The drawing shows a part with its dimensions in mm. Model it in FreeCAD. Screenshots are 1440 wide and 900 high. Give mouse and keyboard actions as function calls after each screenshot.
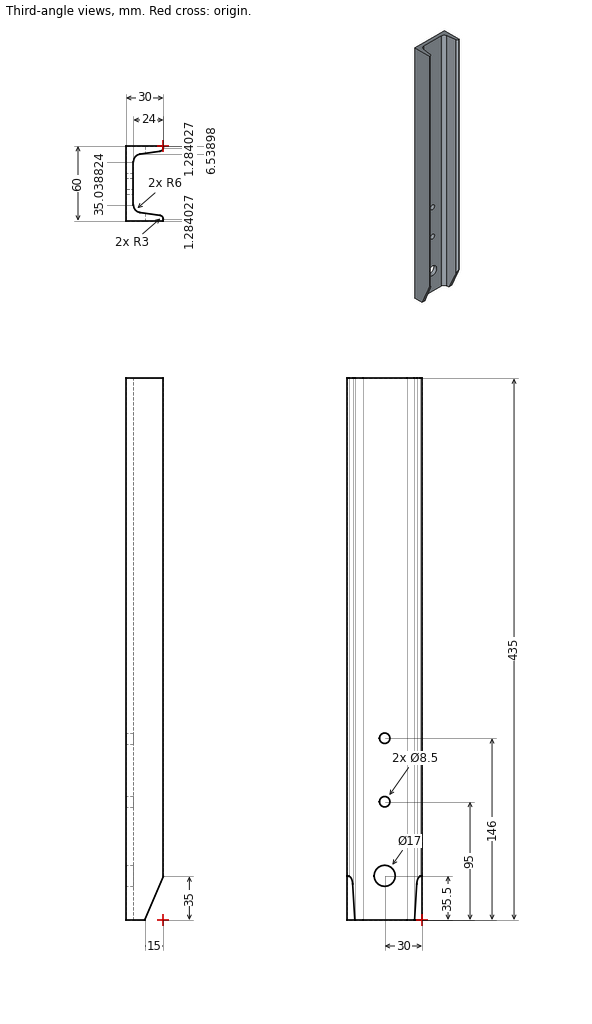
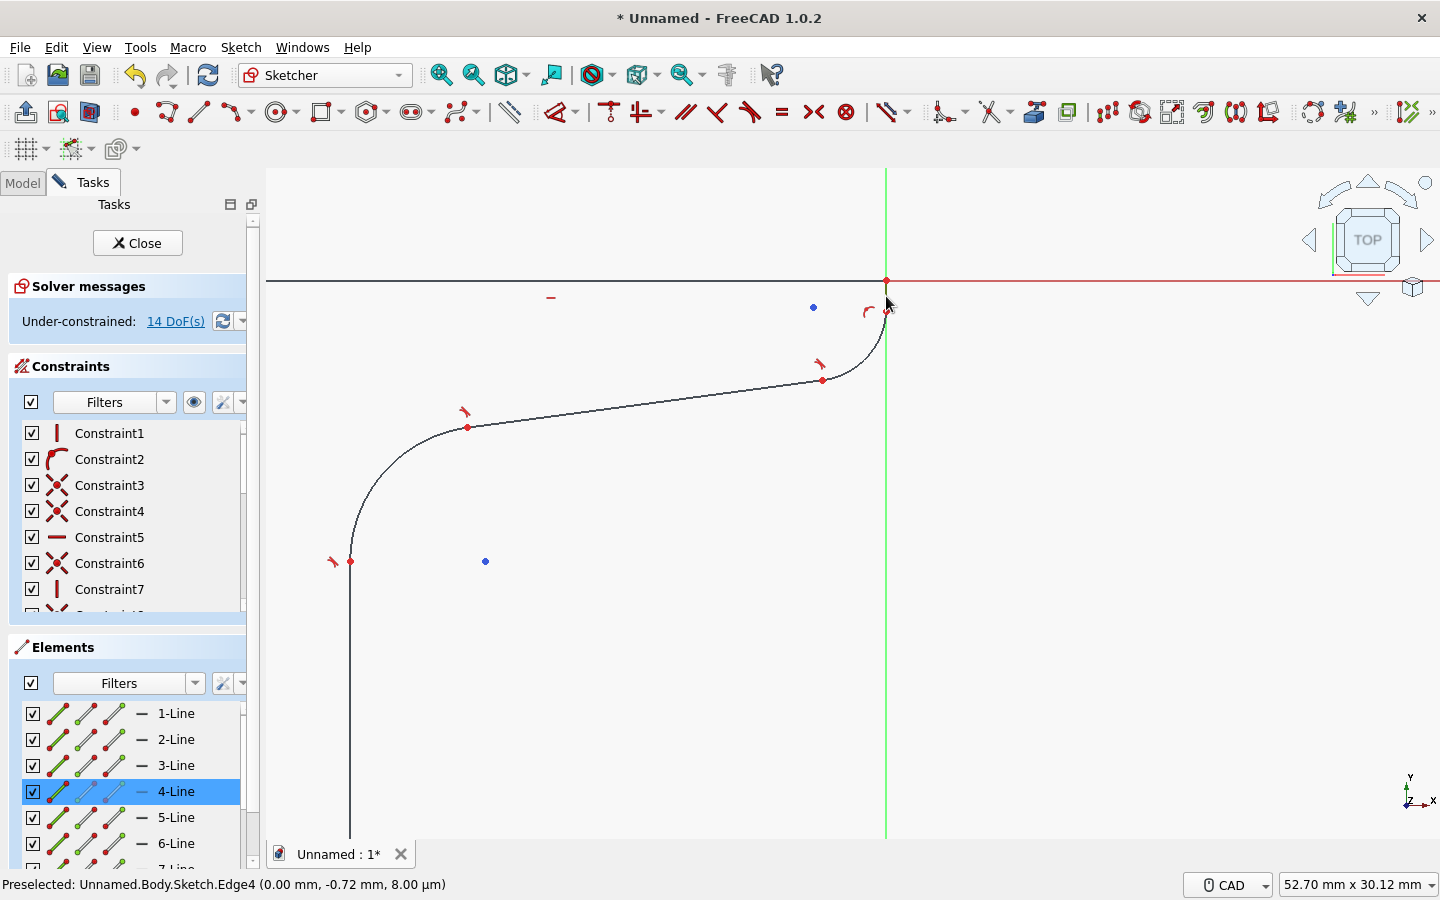
click(851, 370)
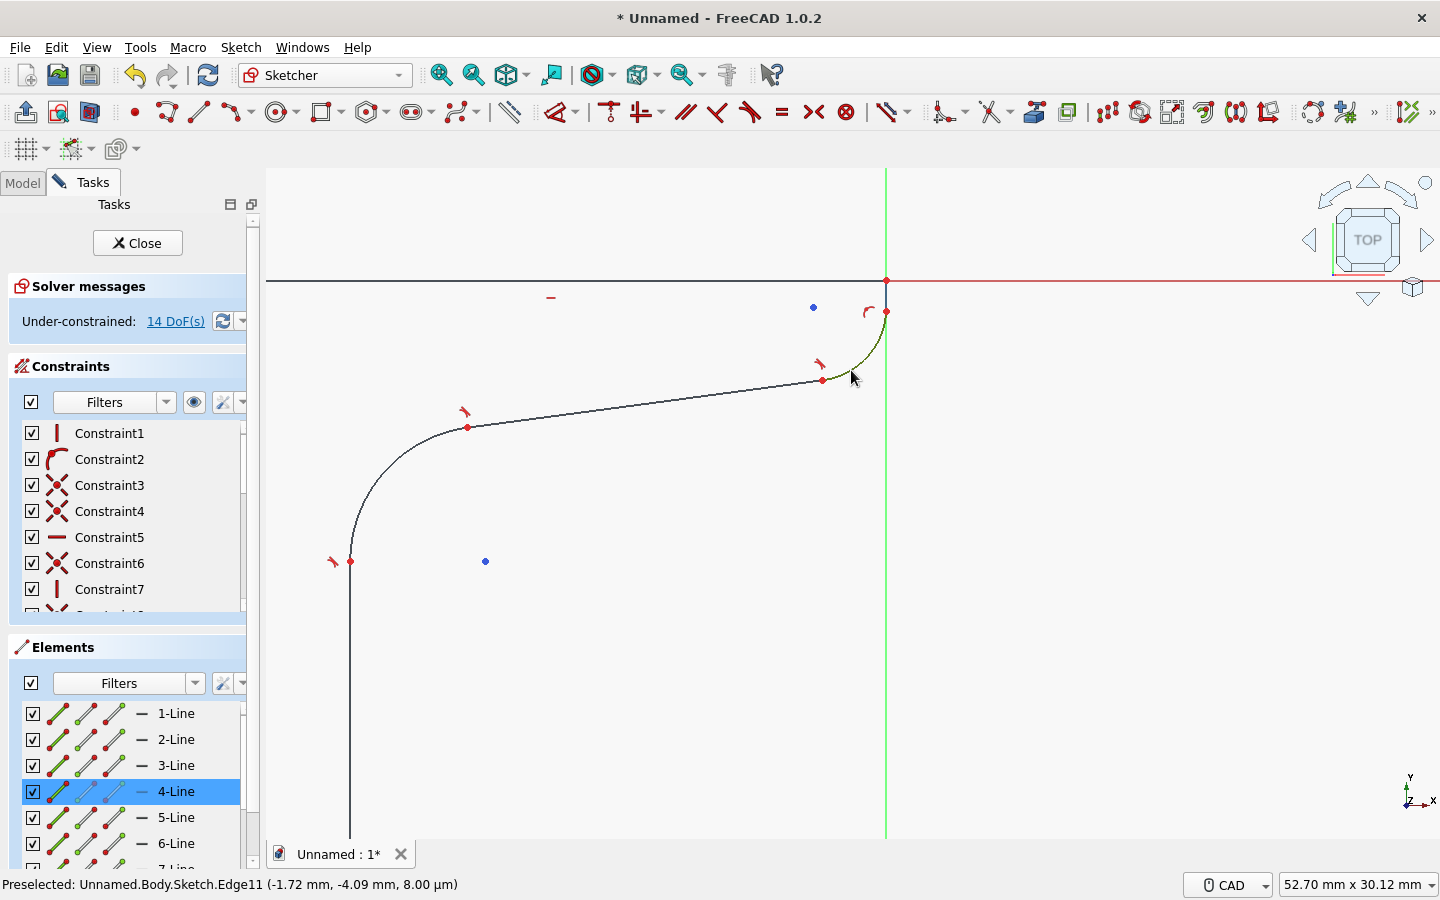
key(t)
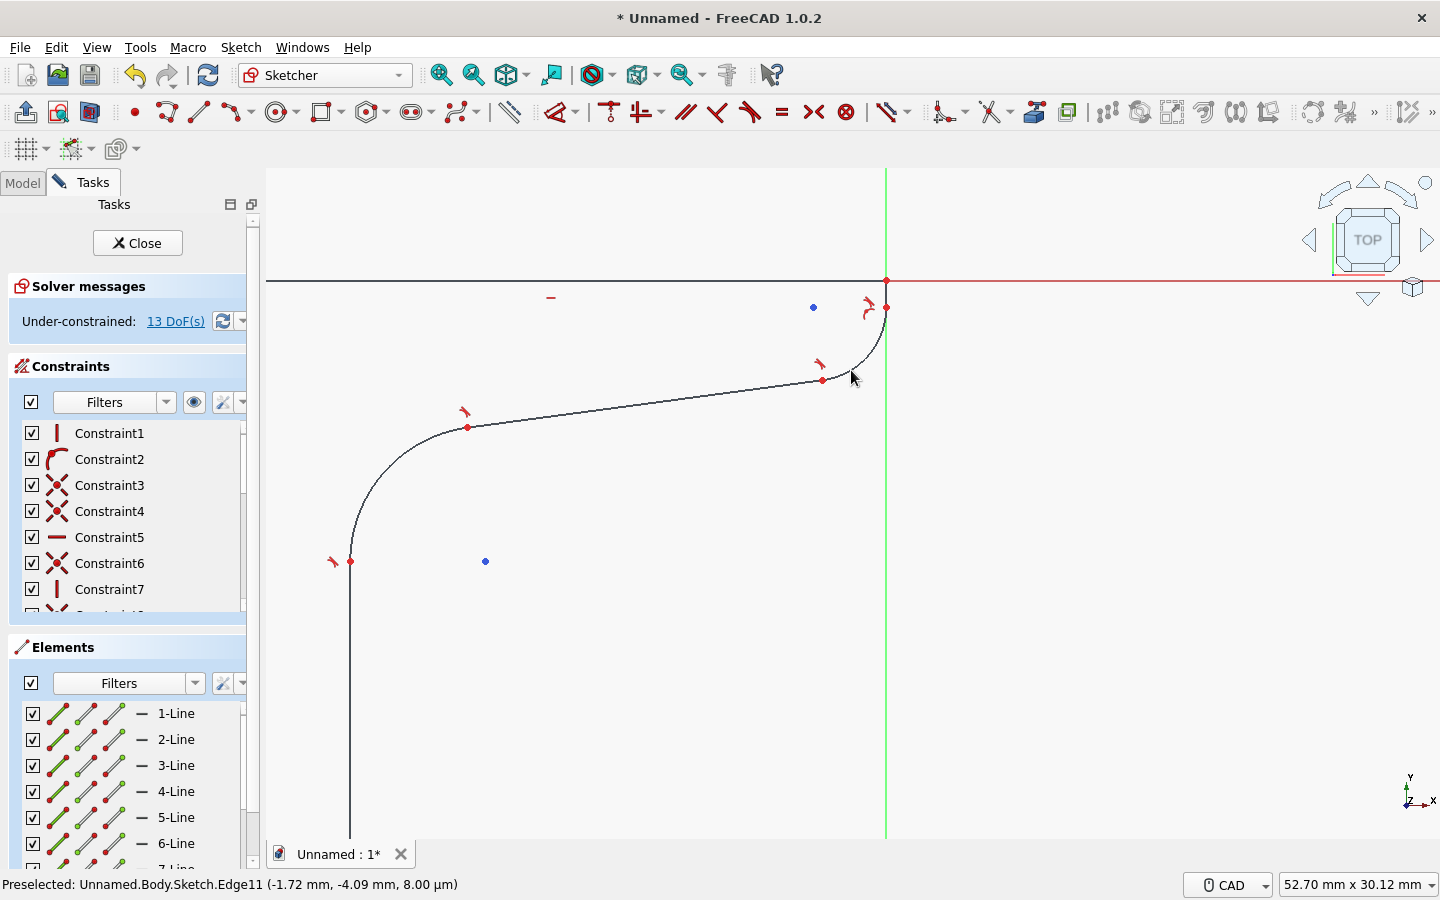
scroll(885, 311, down, 6)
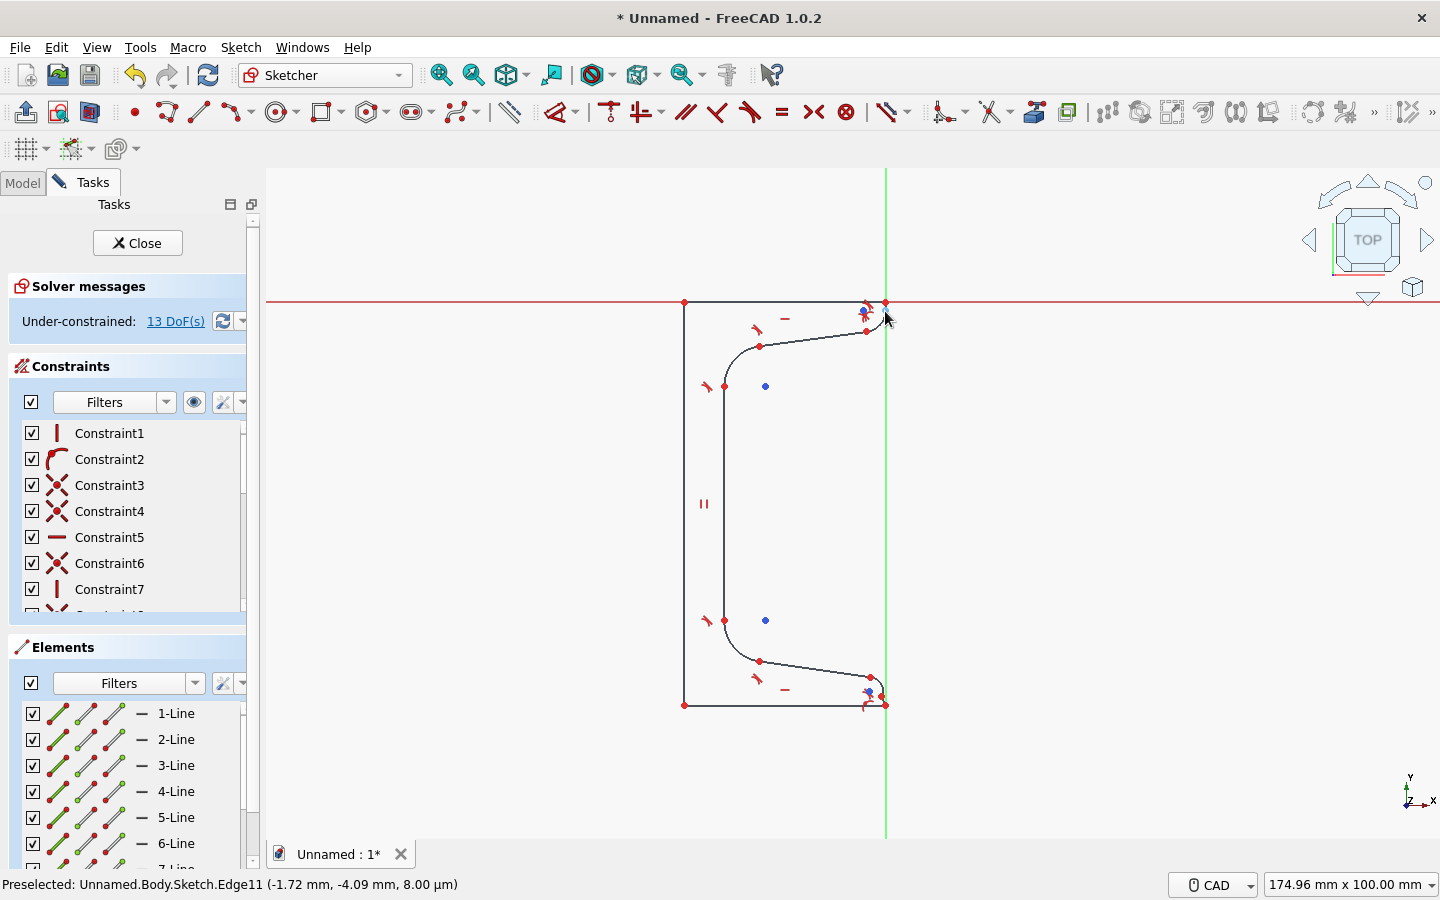
scroll(885, 703, up, 9)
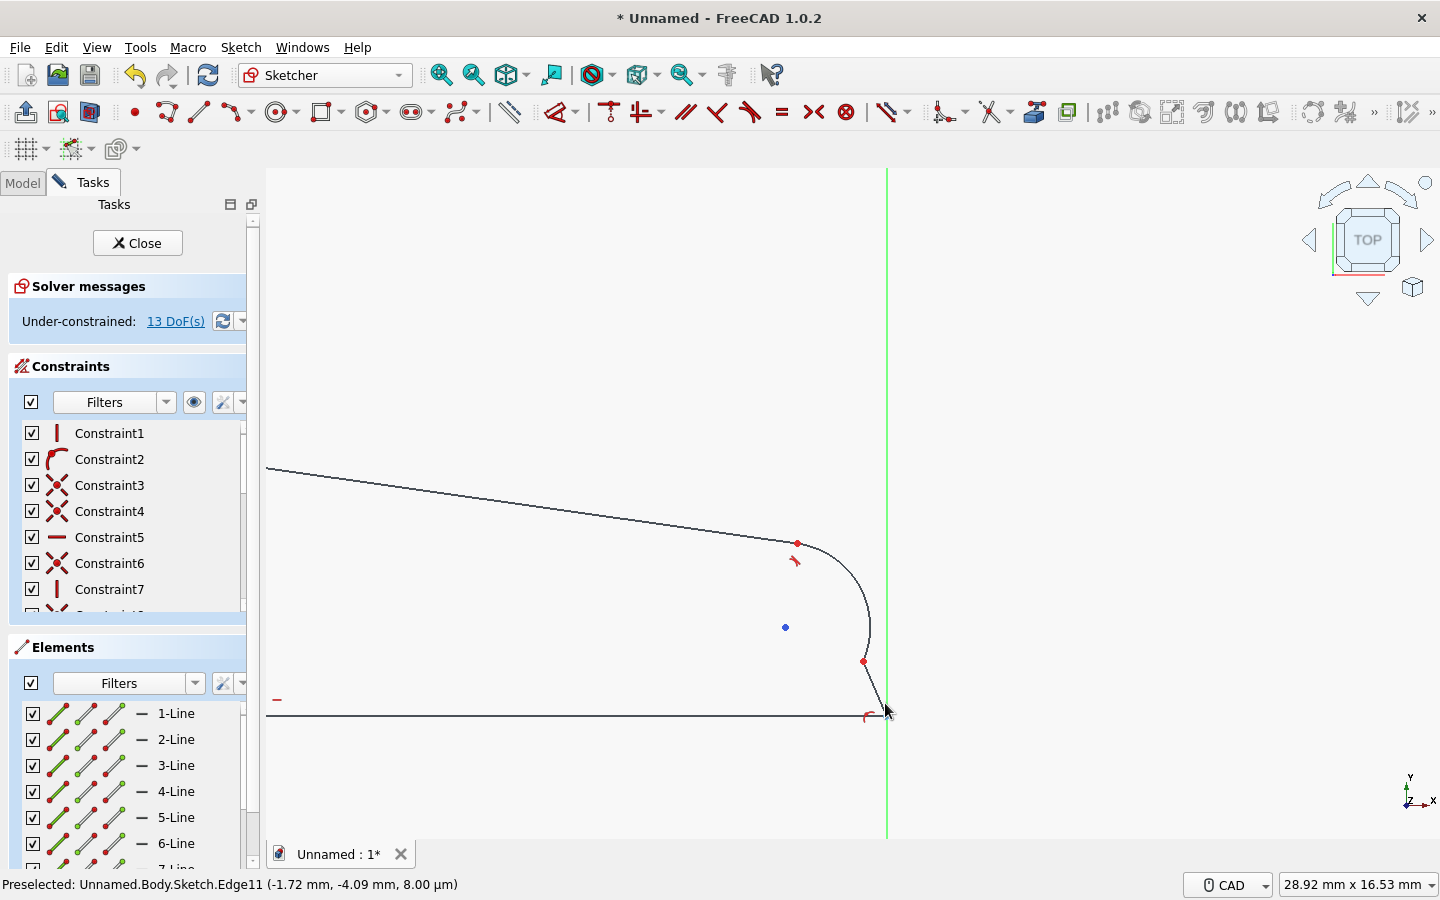
click(880, 700)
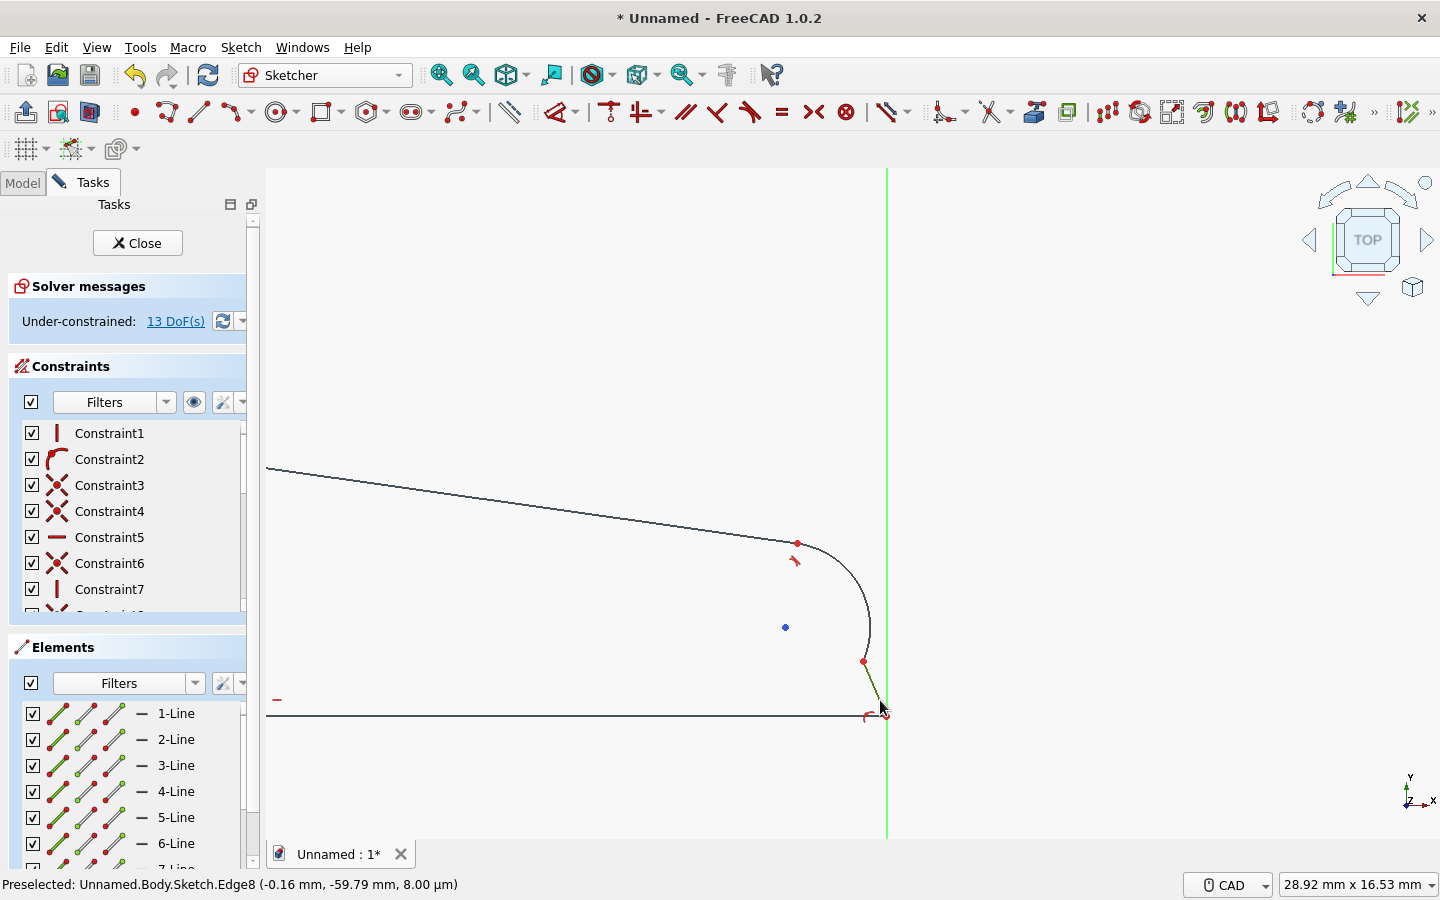
click(869, 616)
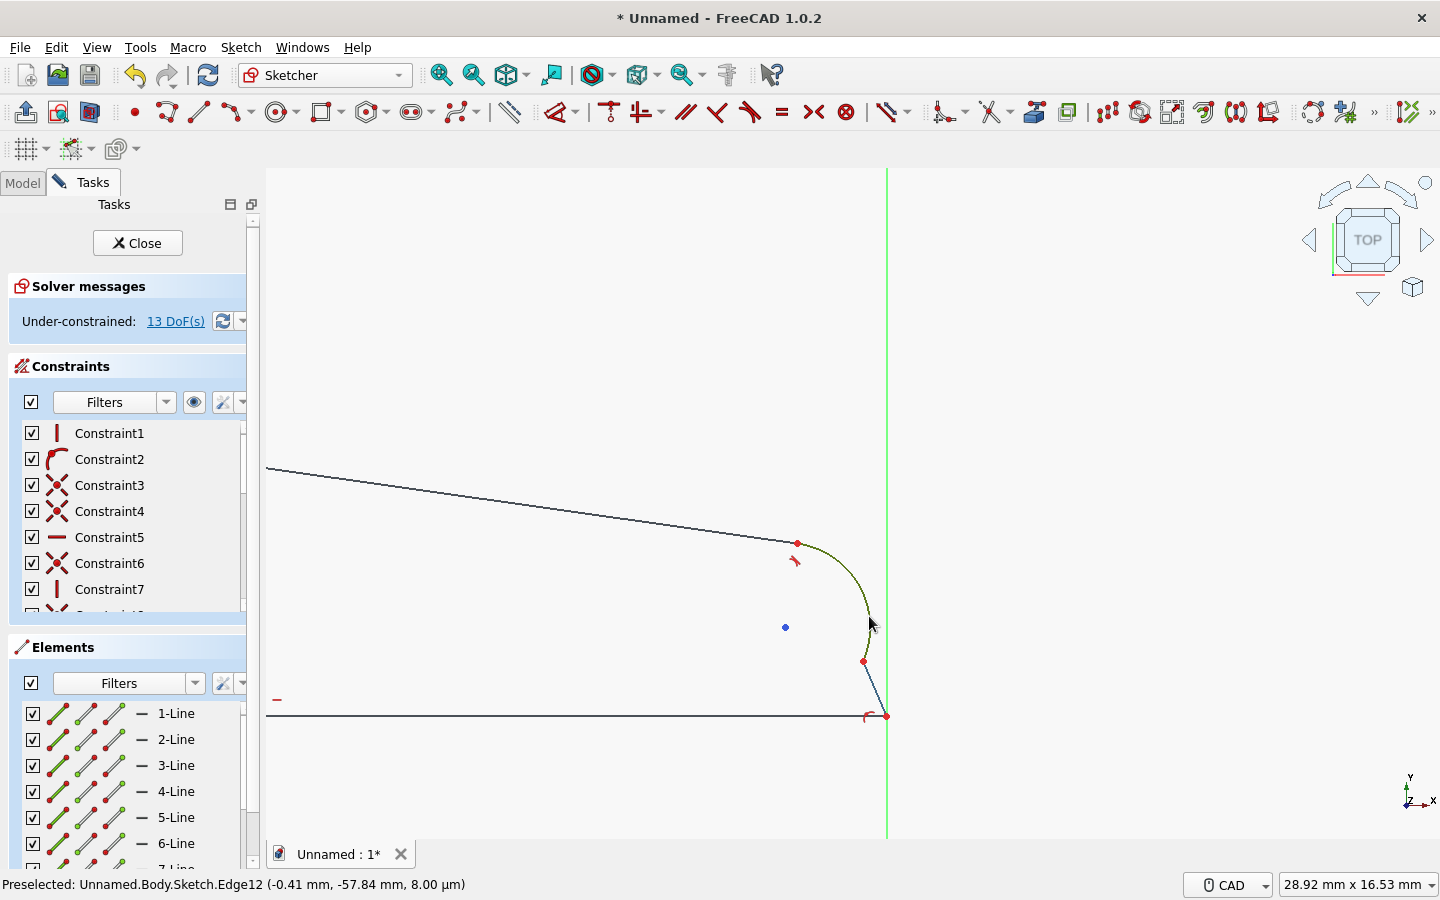
click(750, 112)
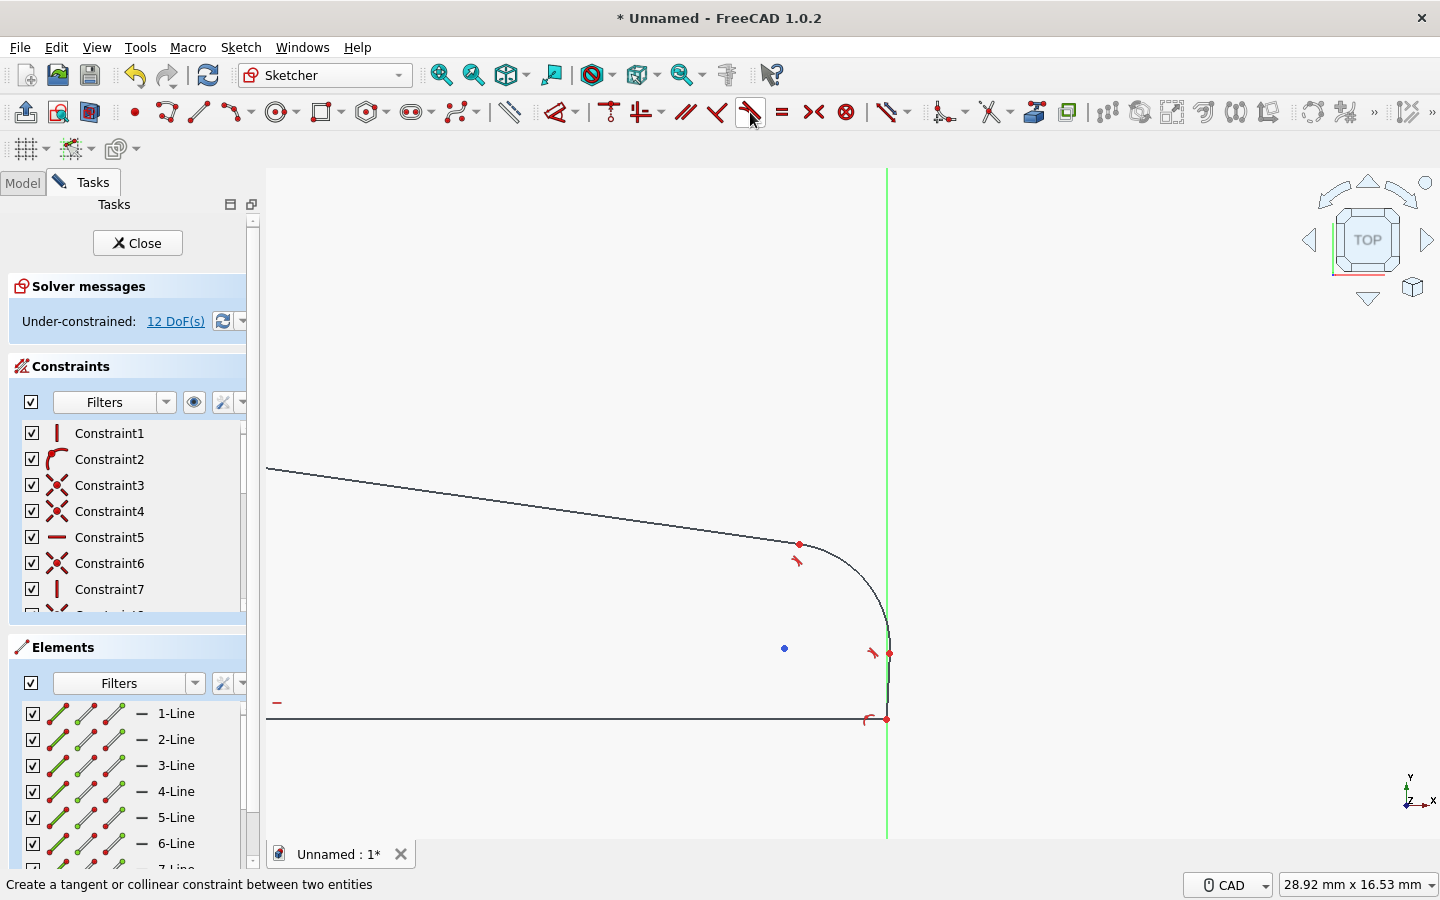
click(888, 700)